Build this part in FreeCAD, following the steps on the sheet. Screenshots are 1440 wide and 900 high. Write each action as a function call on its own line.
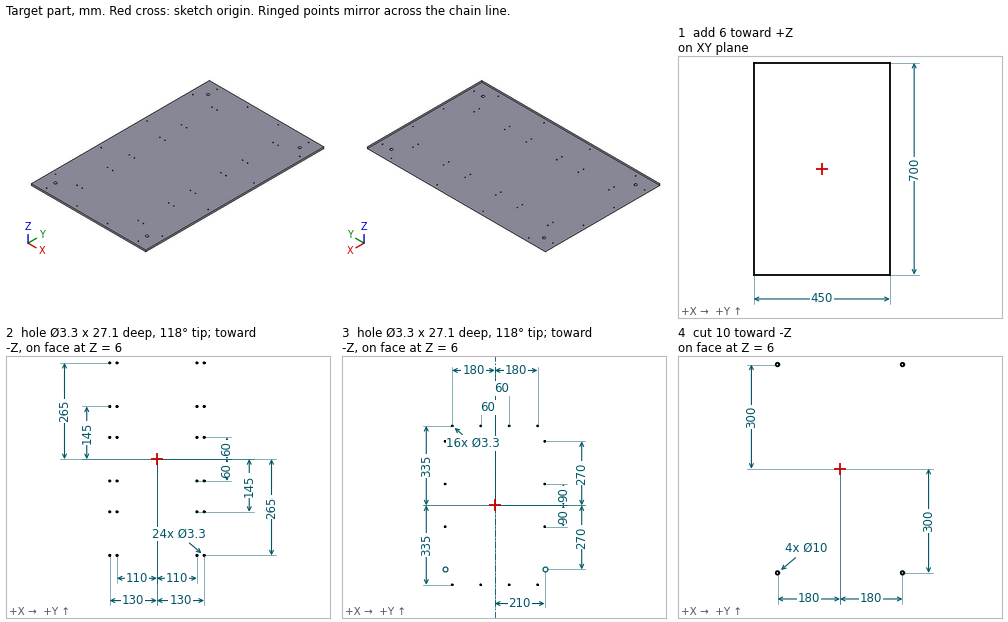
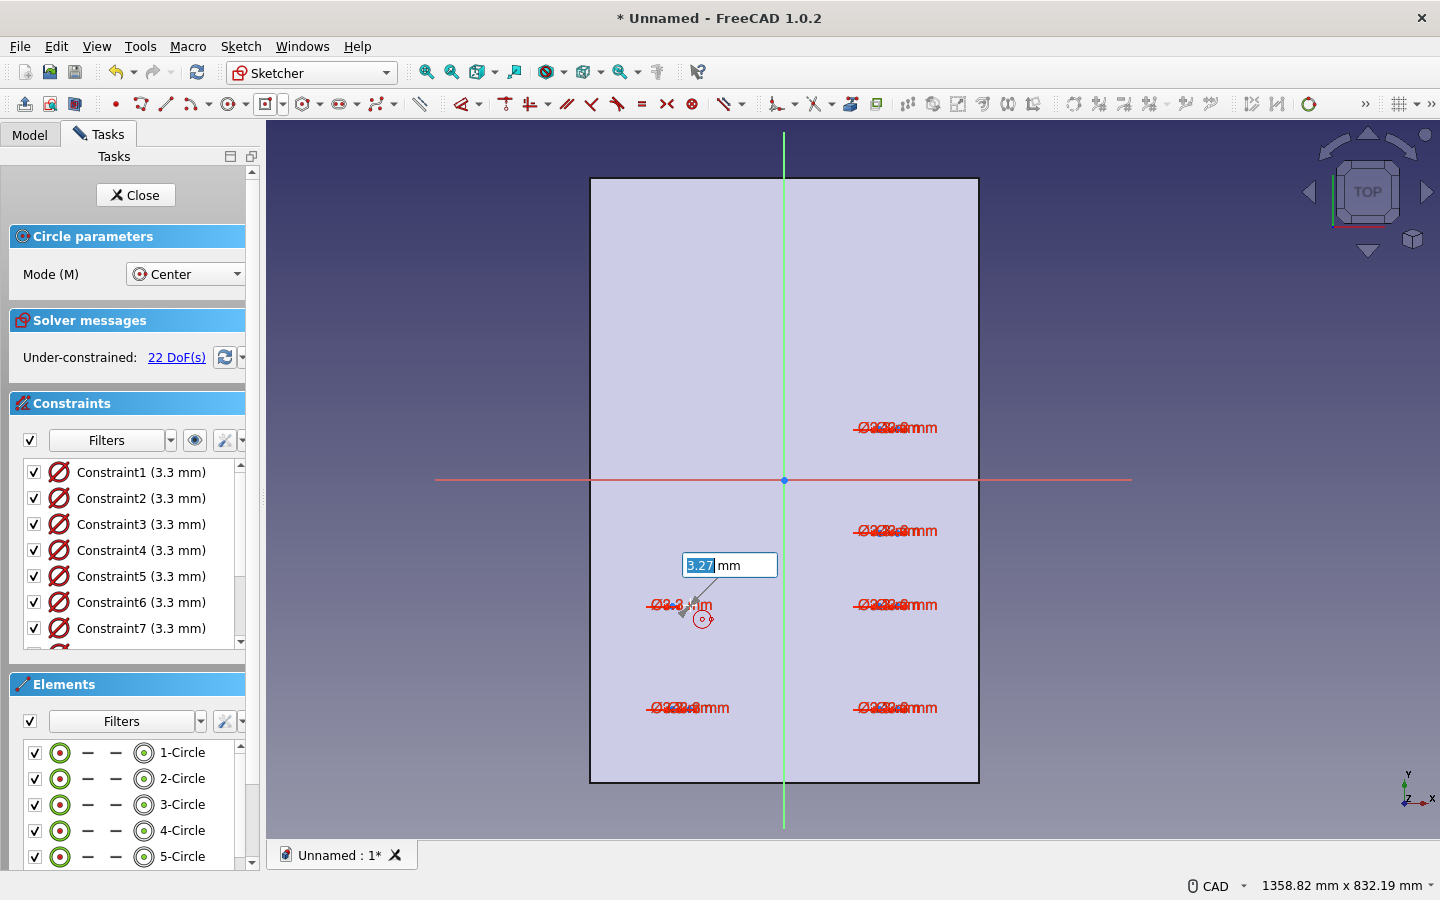
text(3.3)
key(Return)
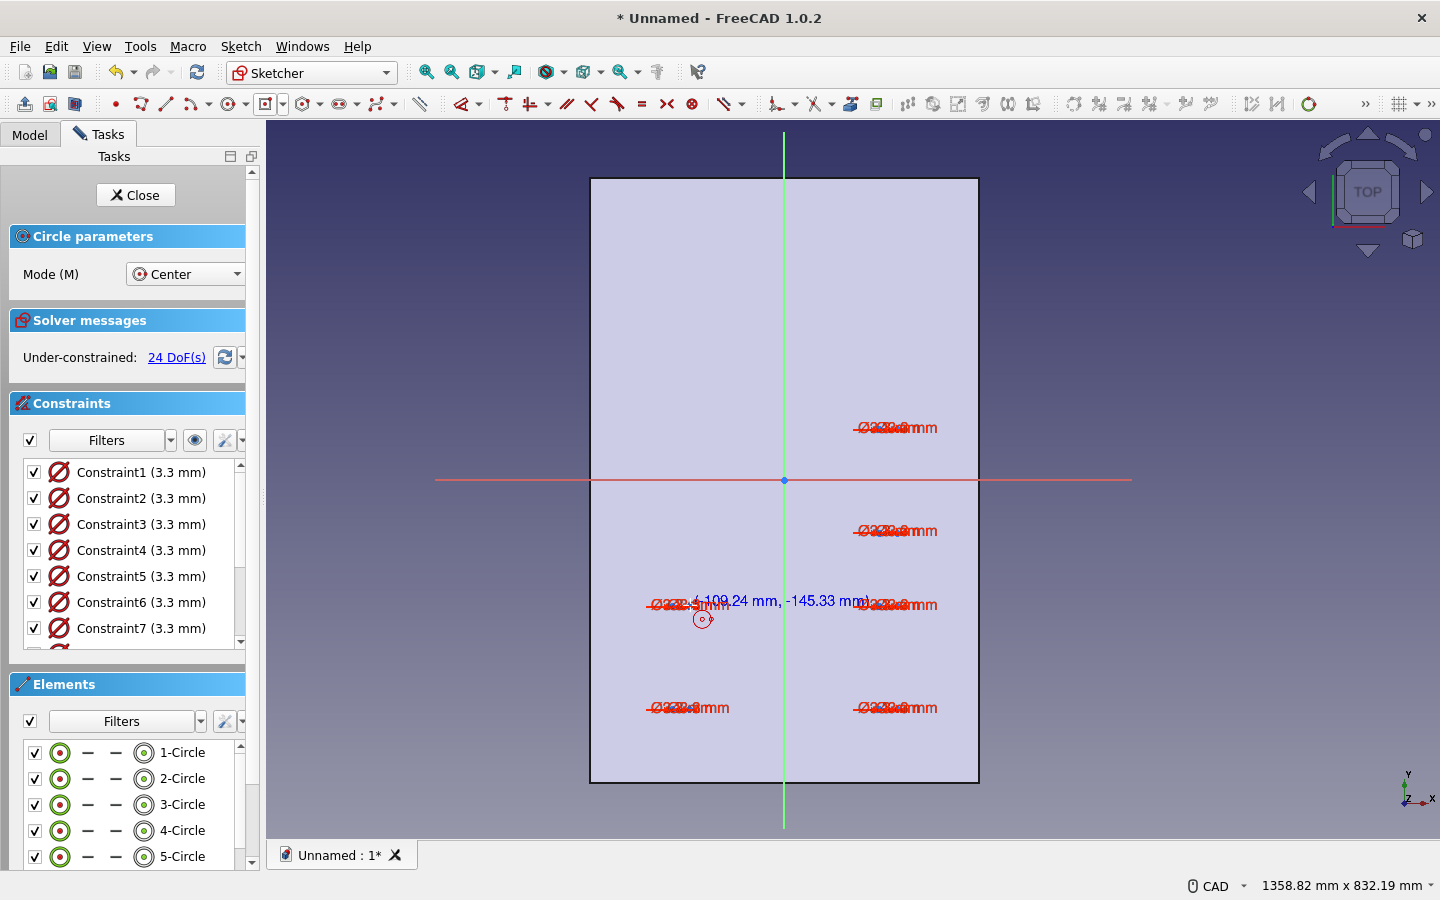
scroll(672, 532, up, 14)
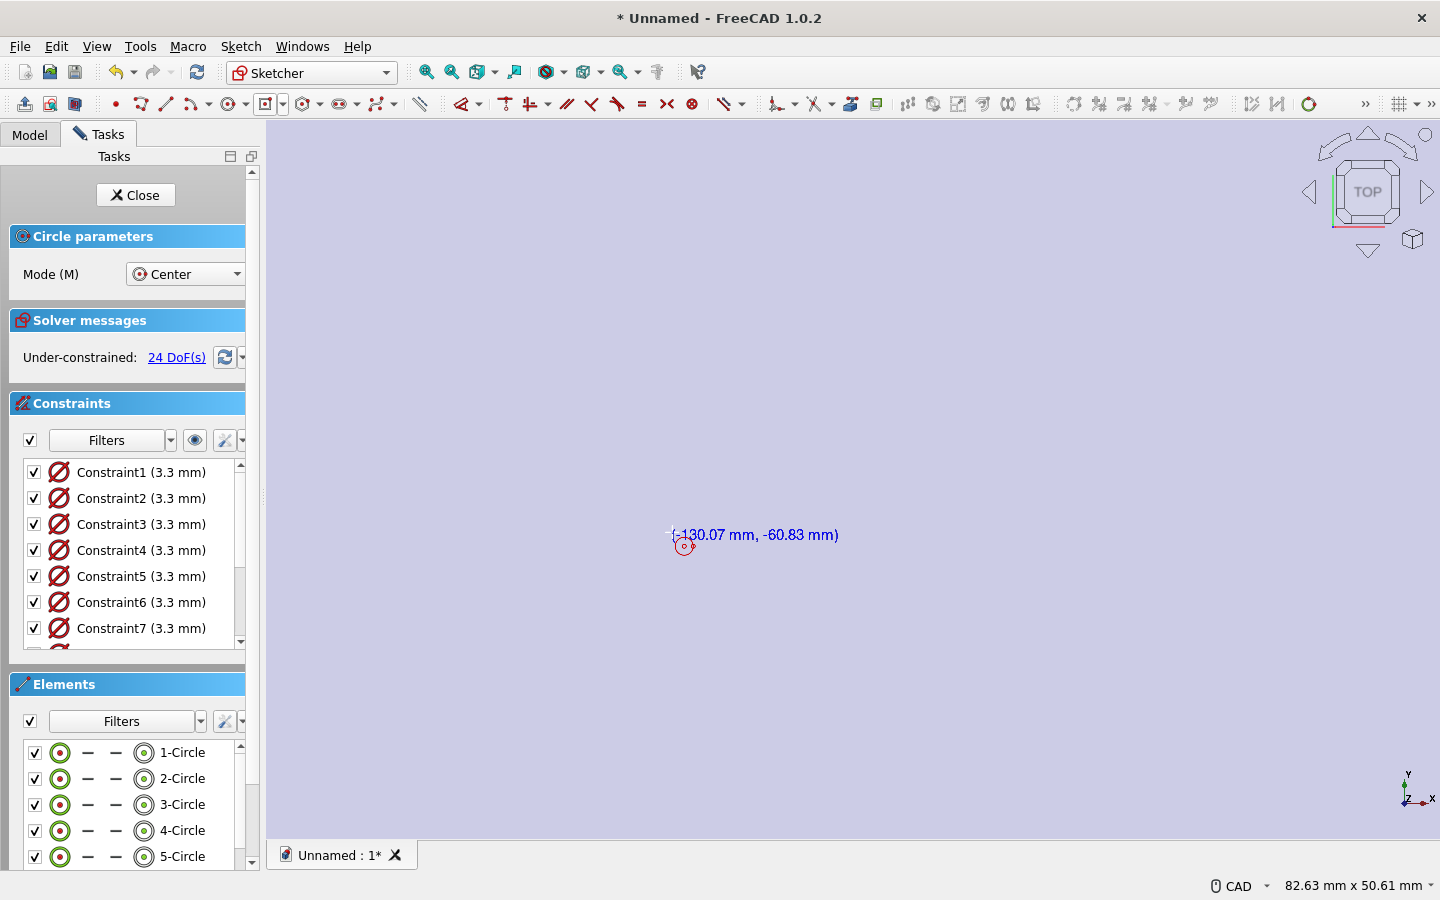
scroll(672, 532, down, 14)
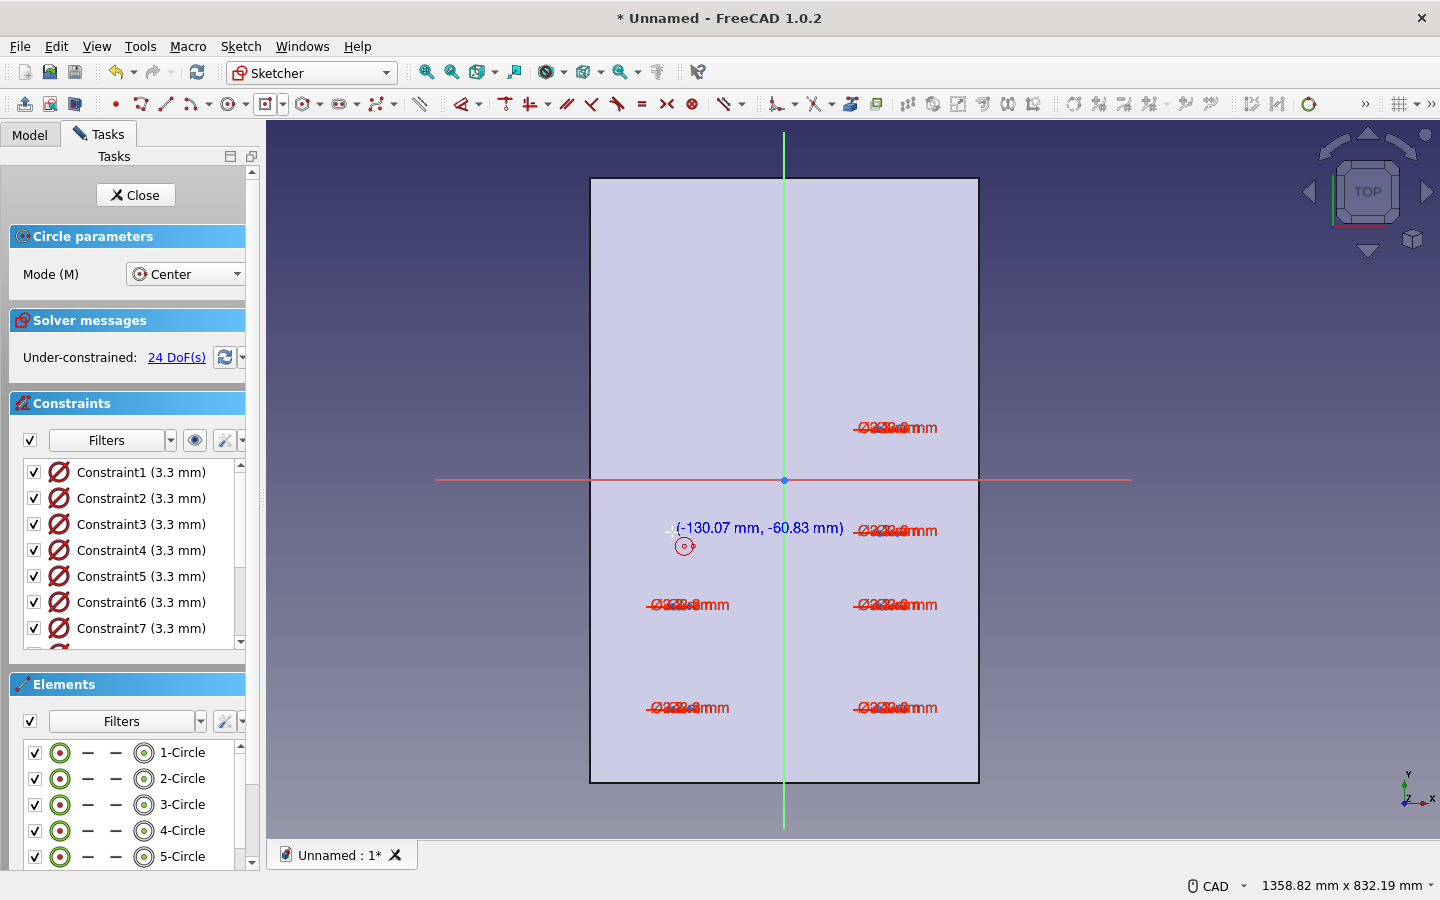
click(672, 532)
move(673, 531)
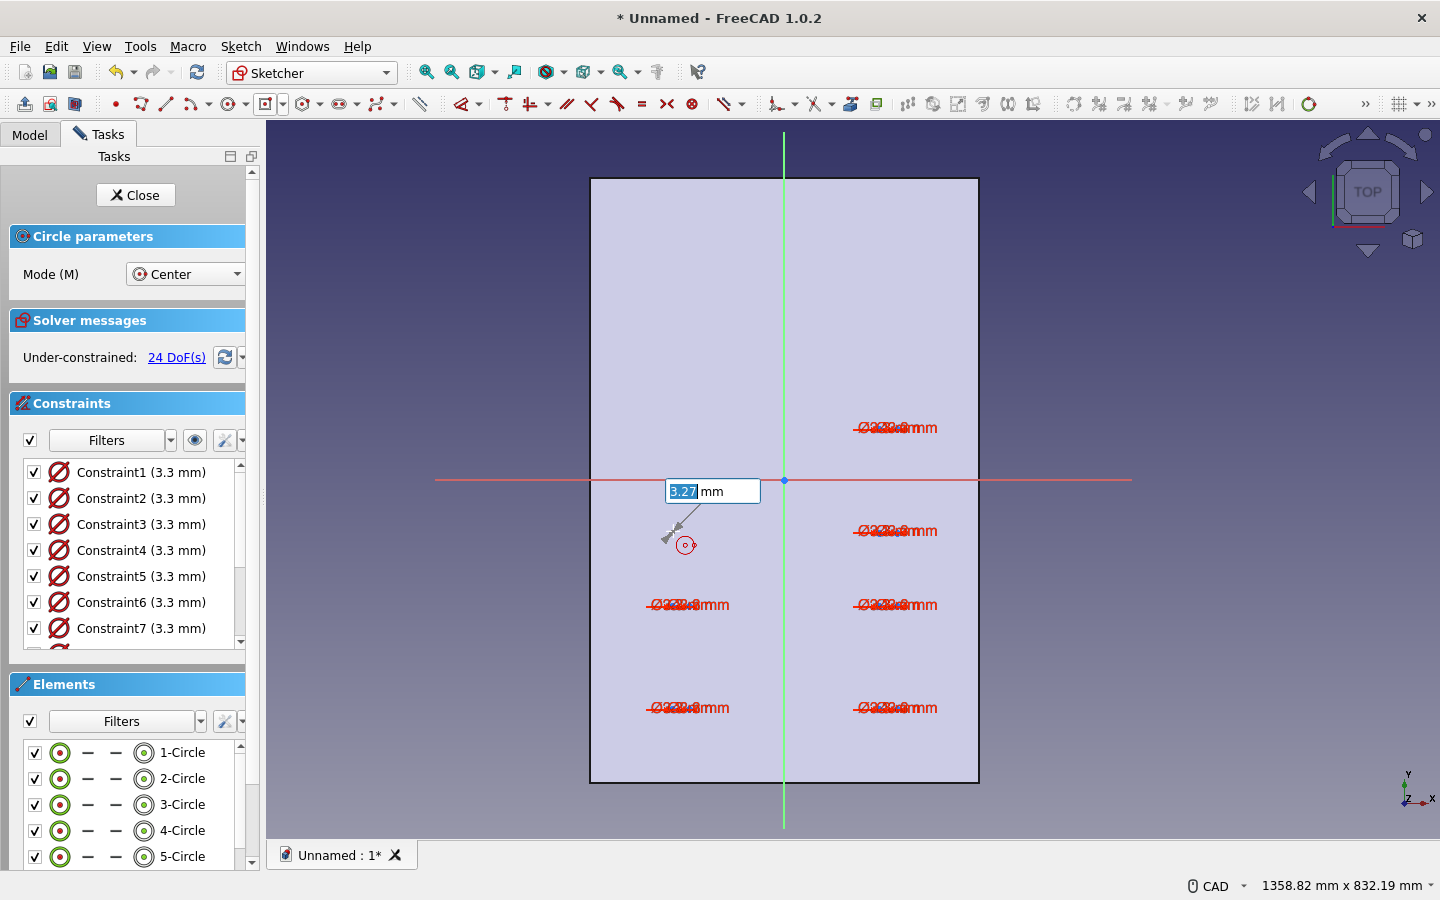
text(3.3)
key(Return)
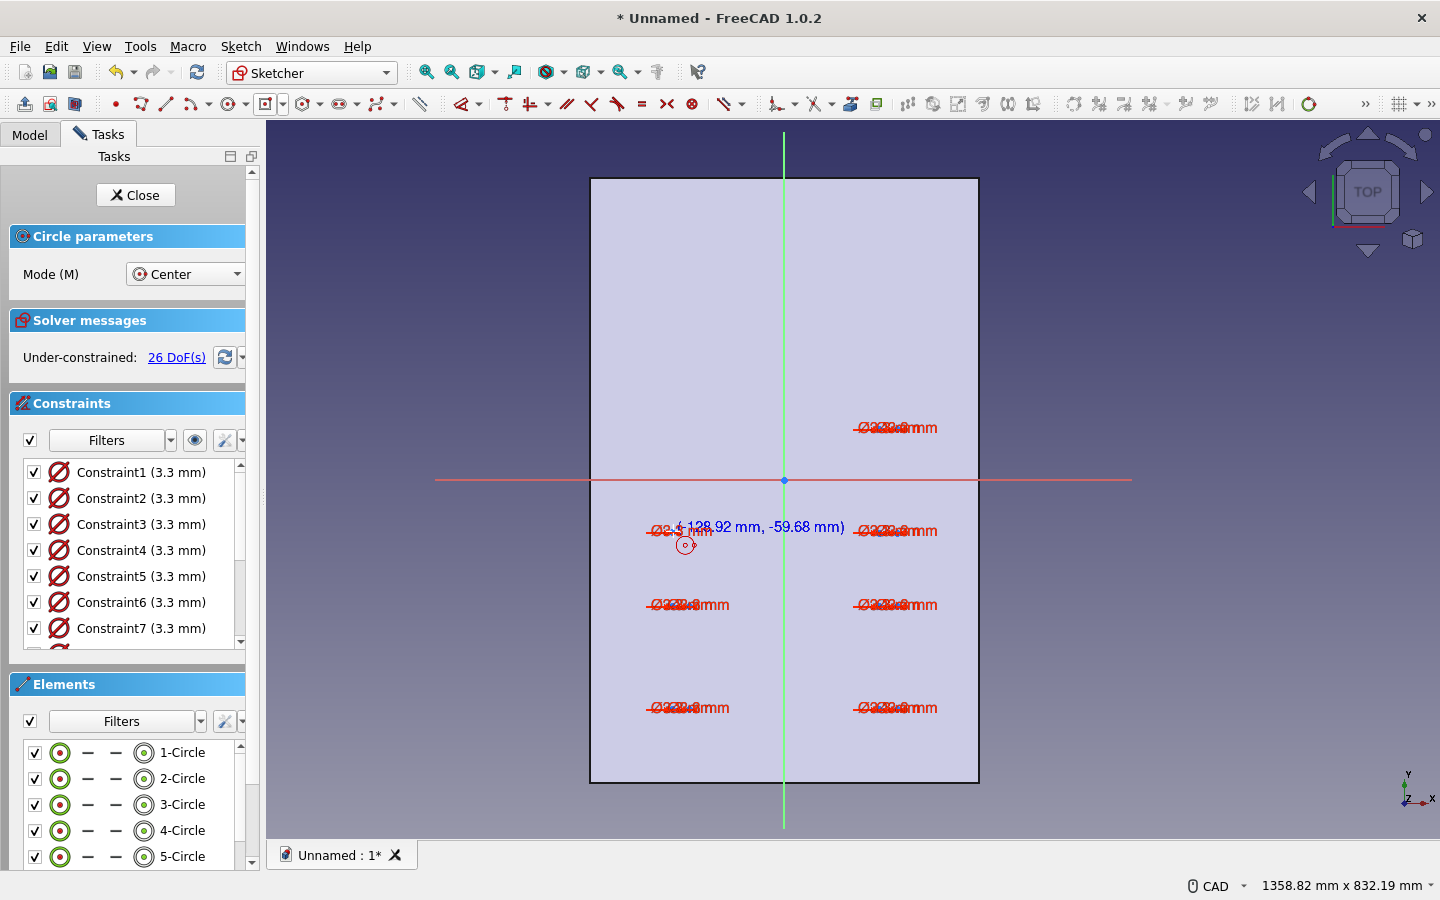
scroll(689, 532, up, 14)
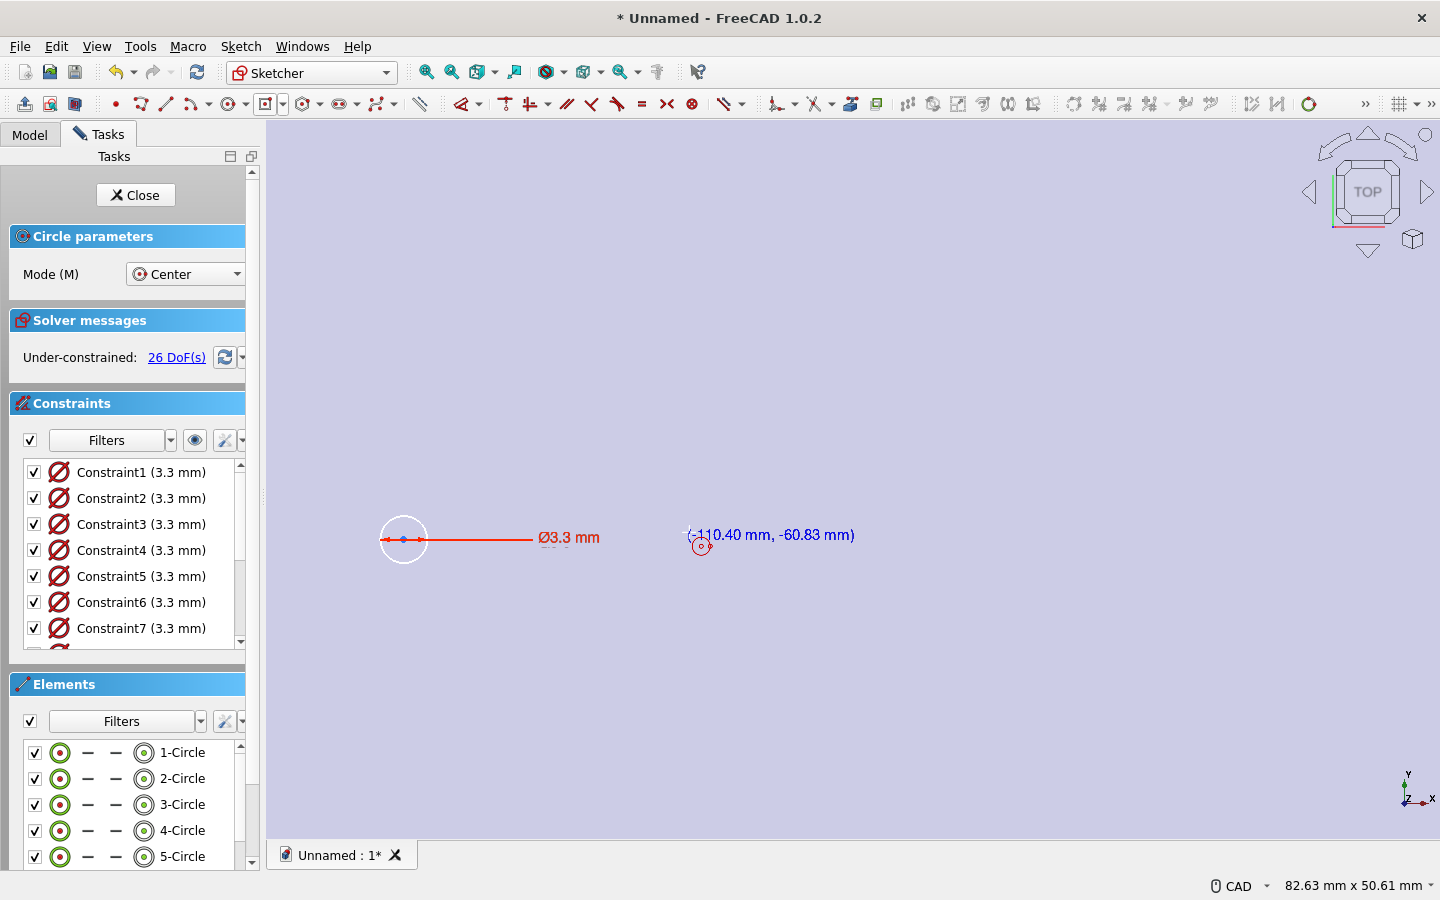
scroll(689, 532, down, 14)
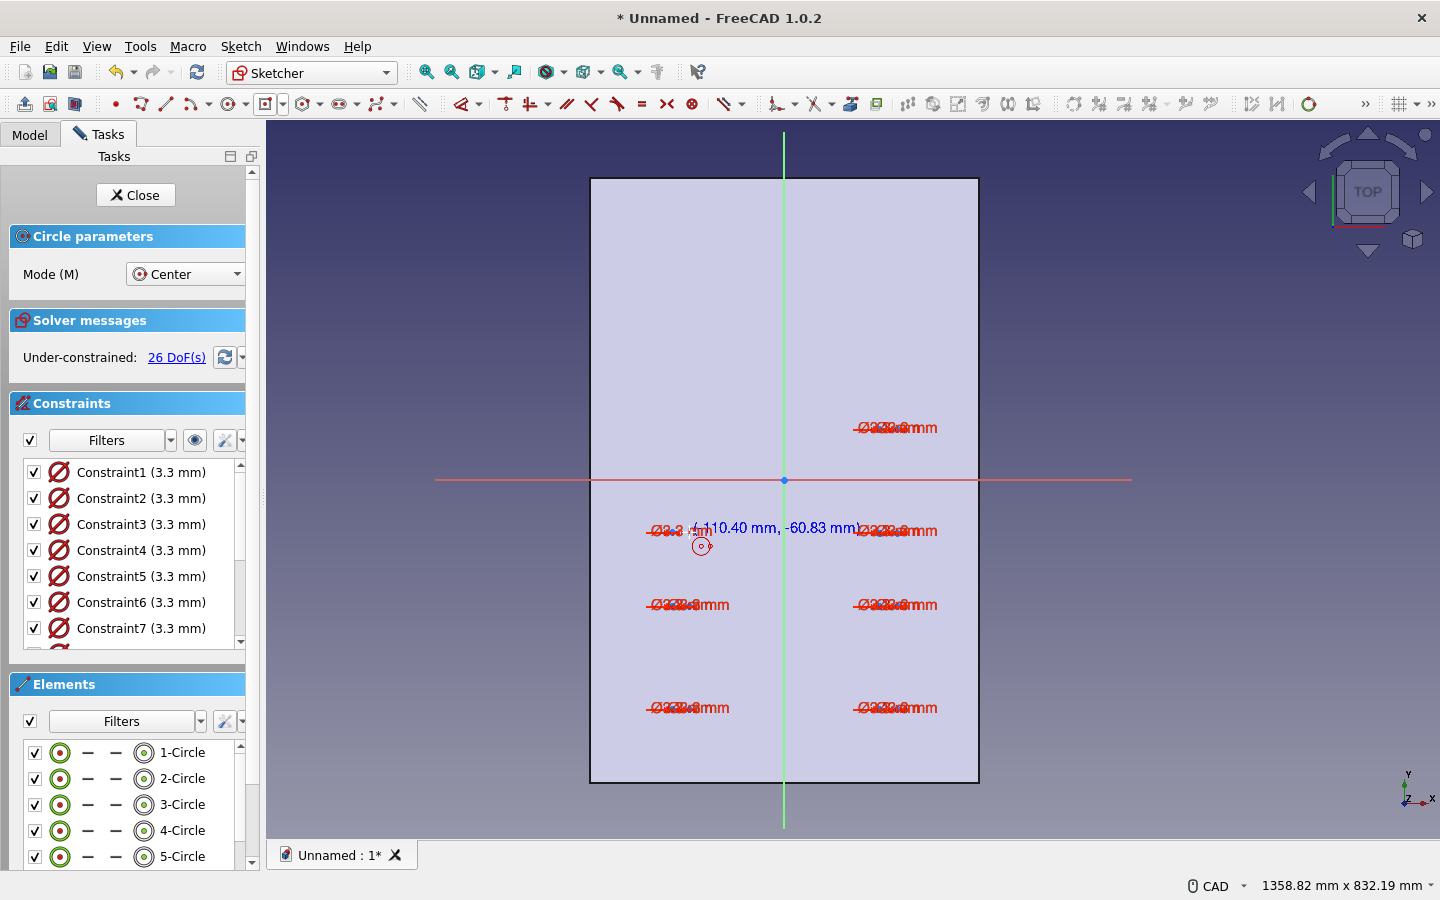
click(689, 532)
move(690, 531)